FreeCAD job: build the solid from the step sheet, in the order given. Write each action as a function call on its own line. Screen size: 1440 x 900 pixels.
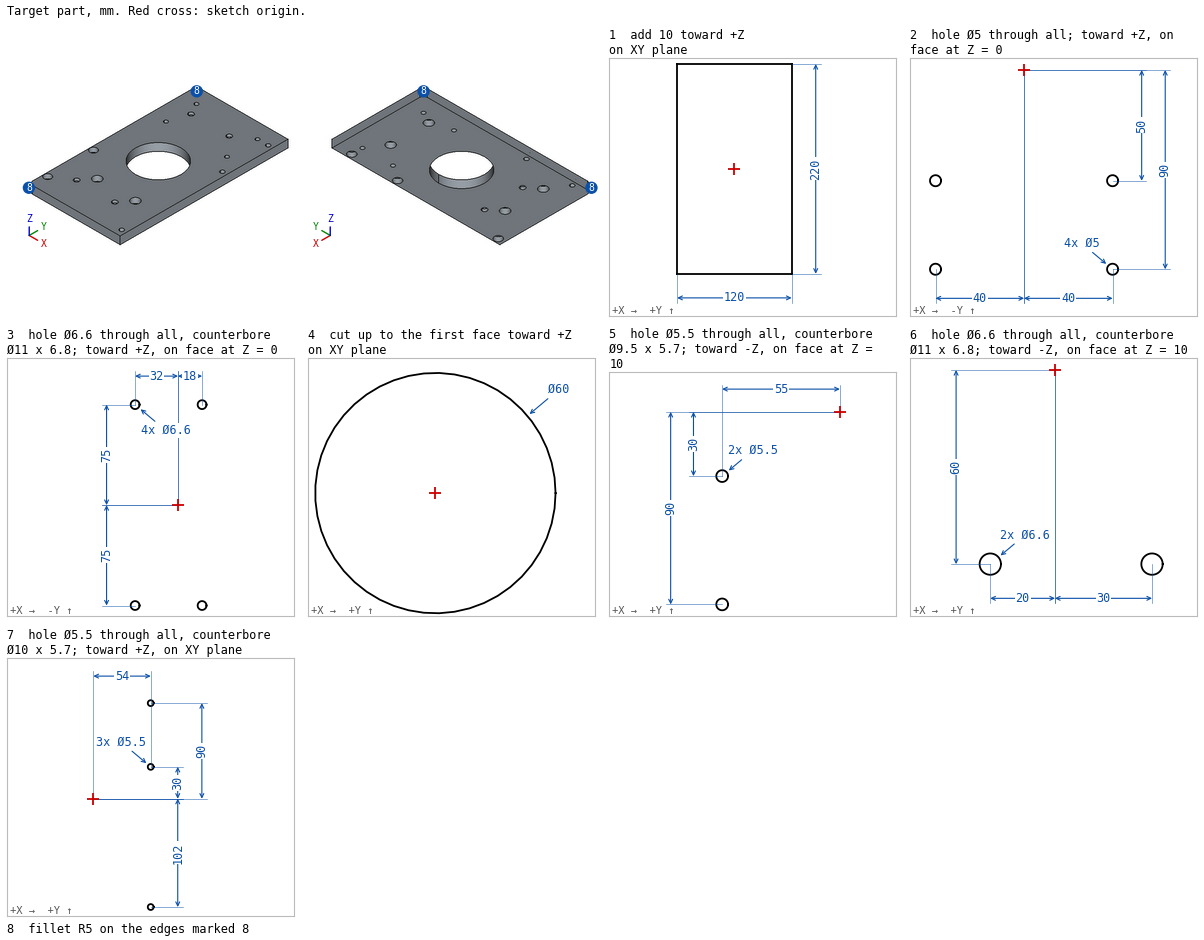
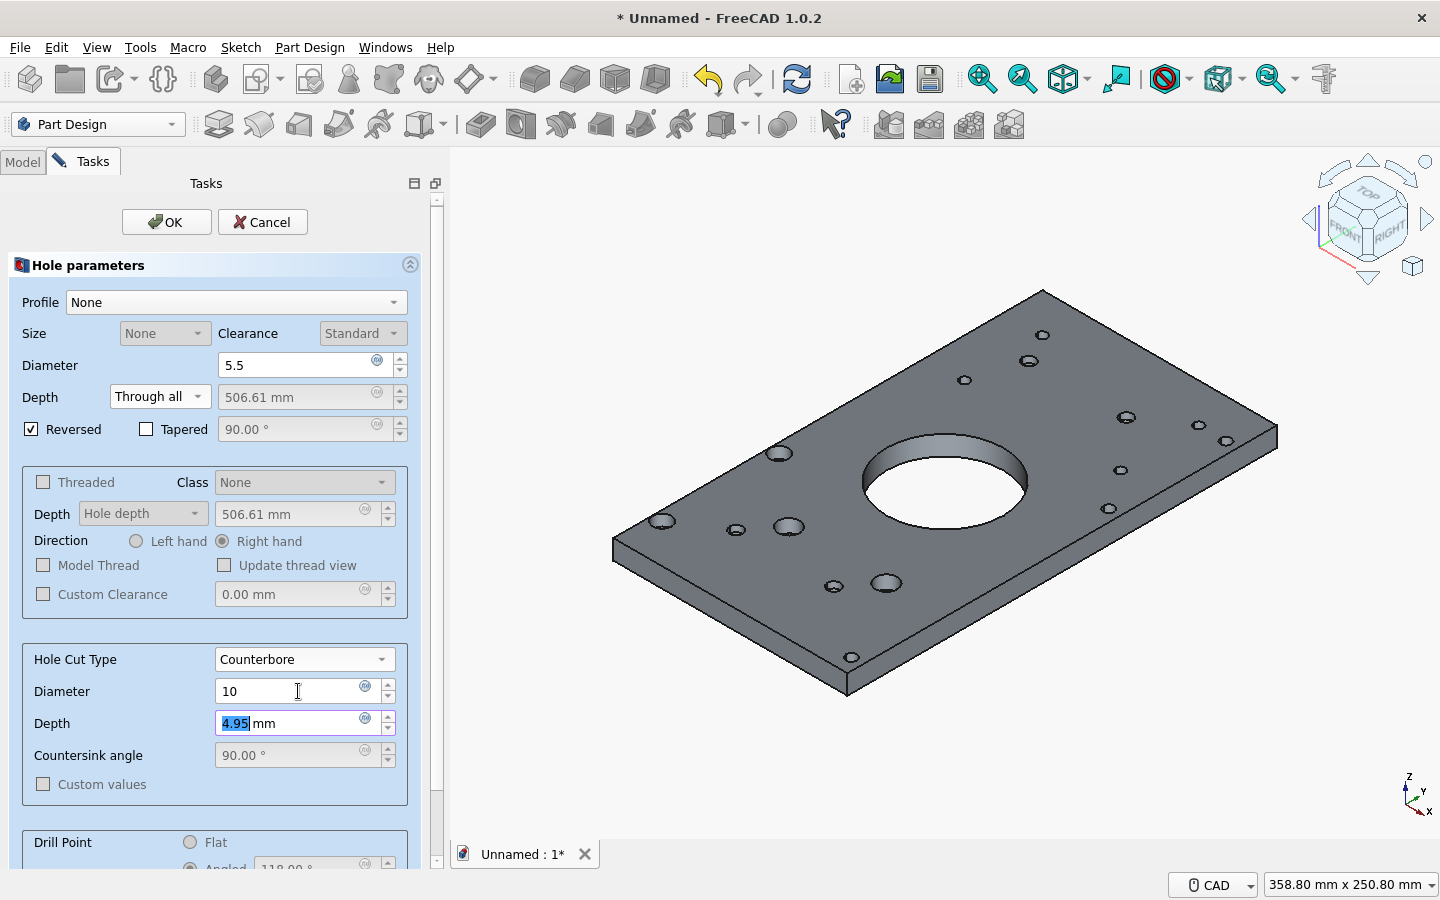
text(5.7)
key(Tab)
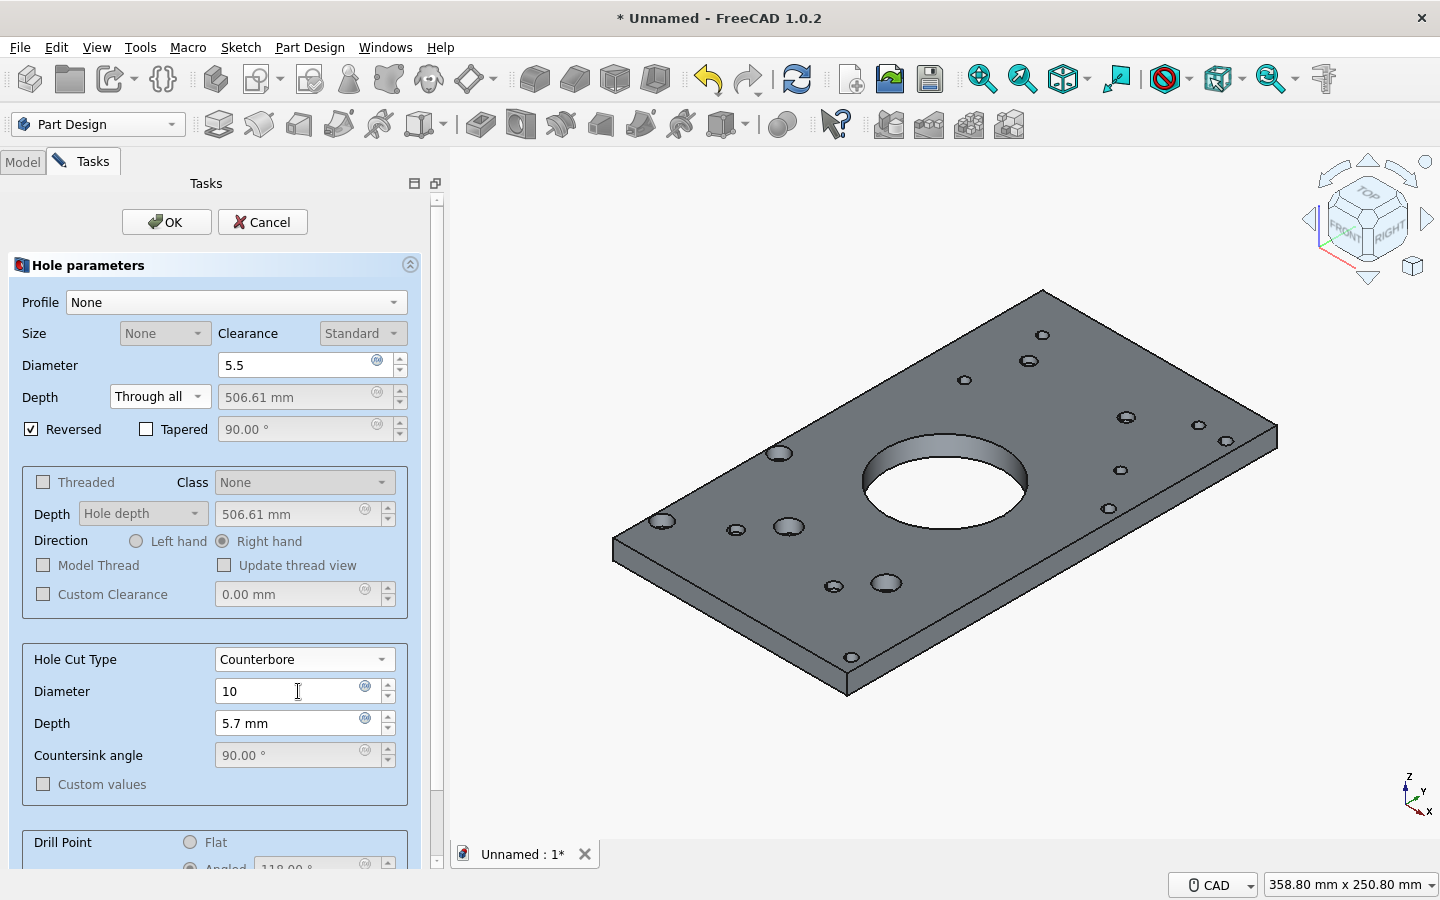
click(167, 222)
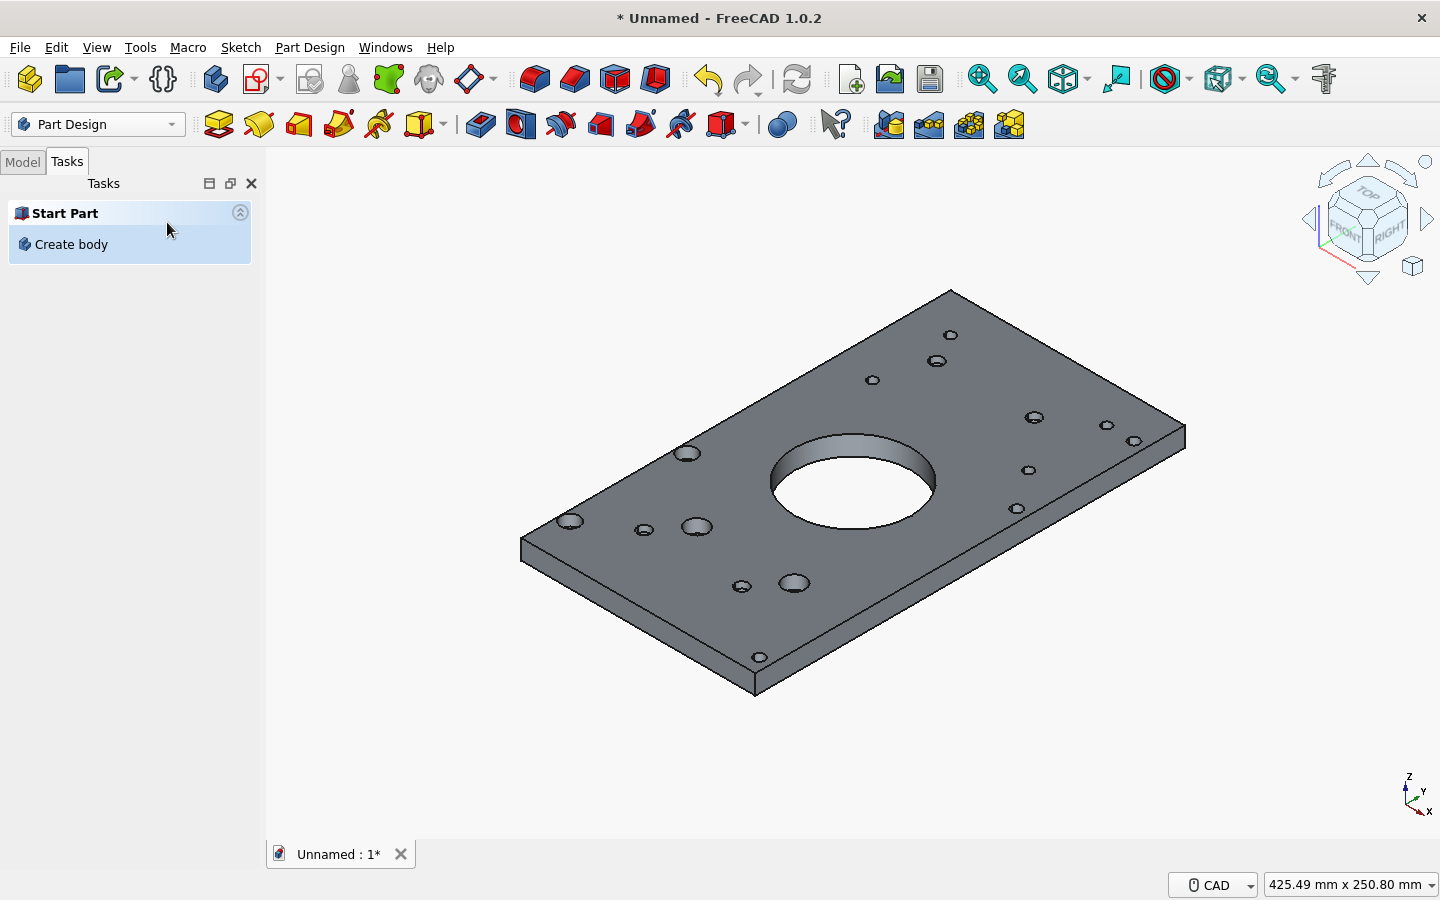
key(2)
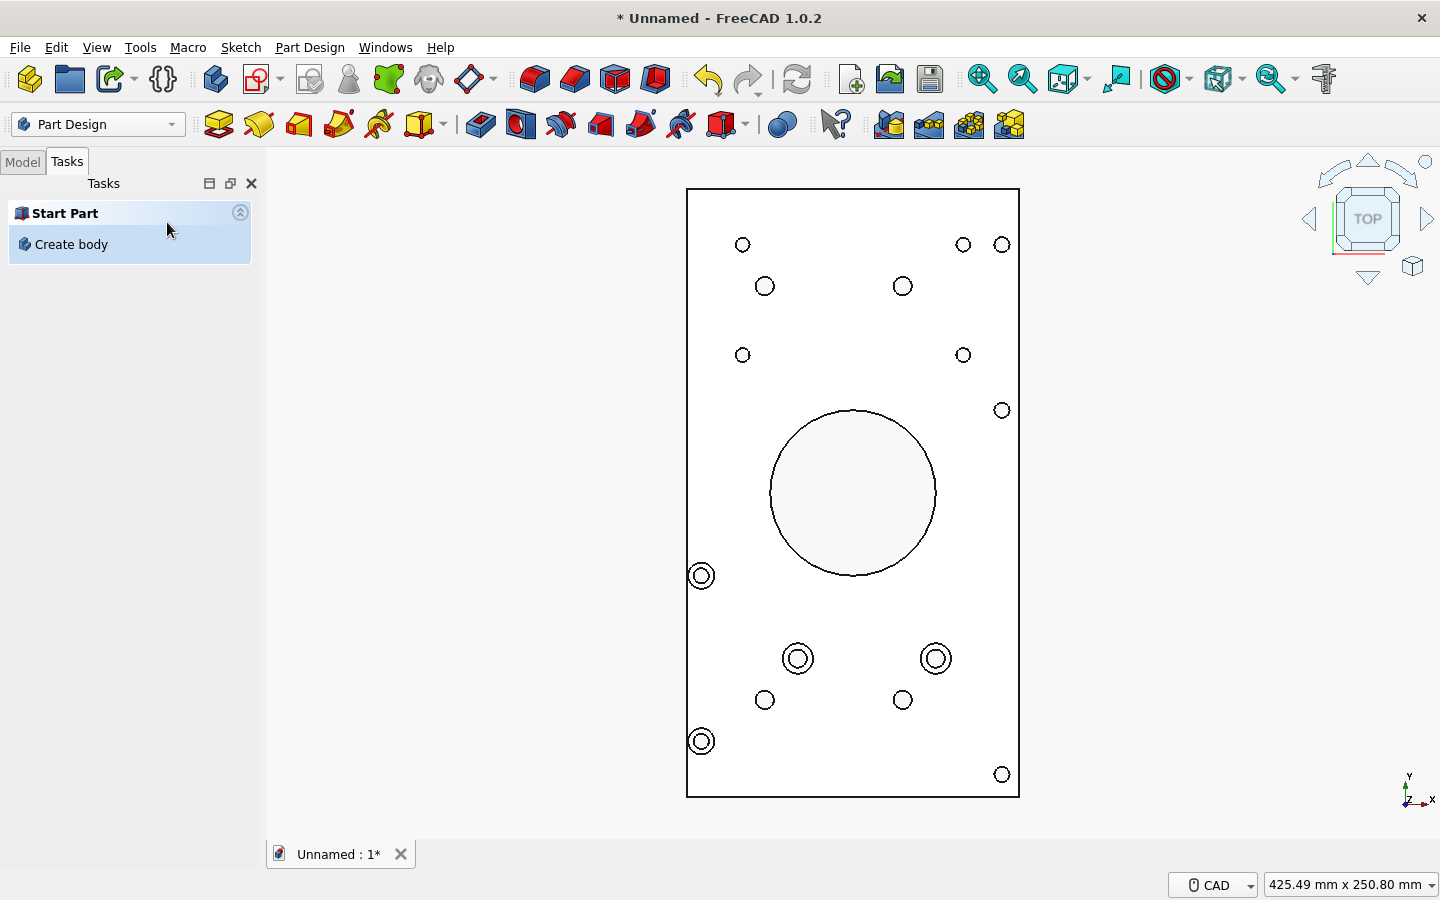
key(0)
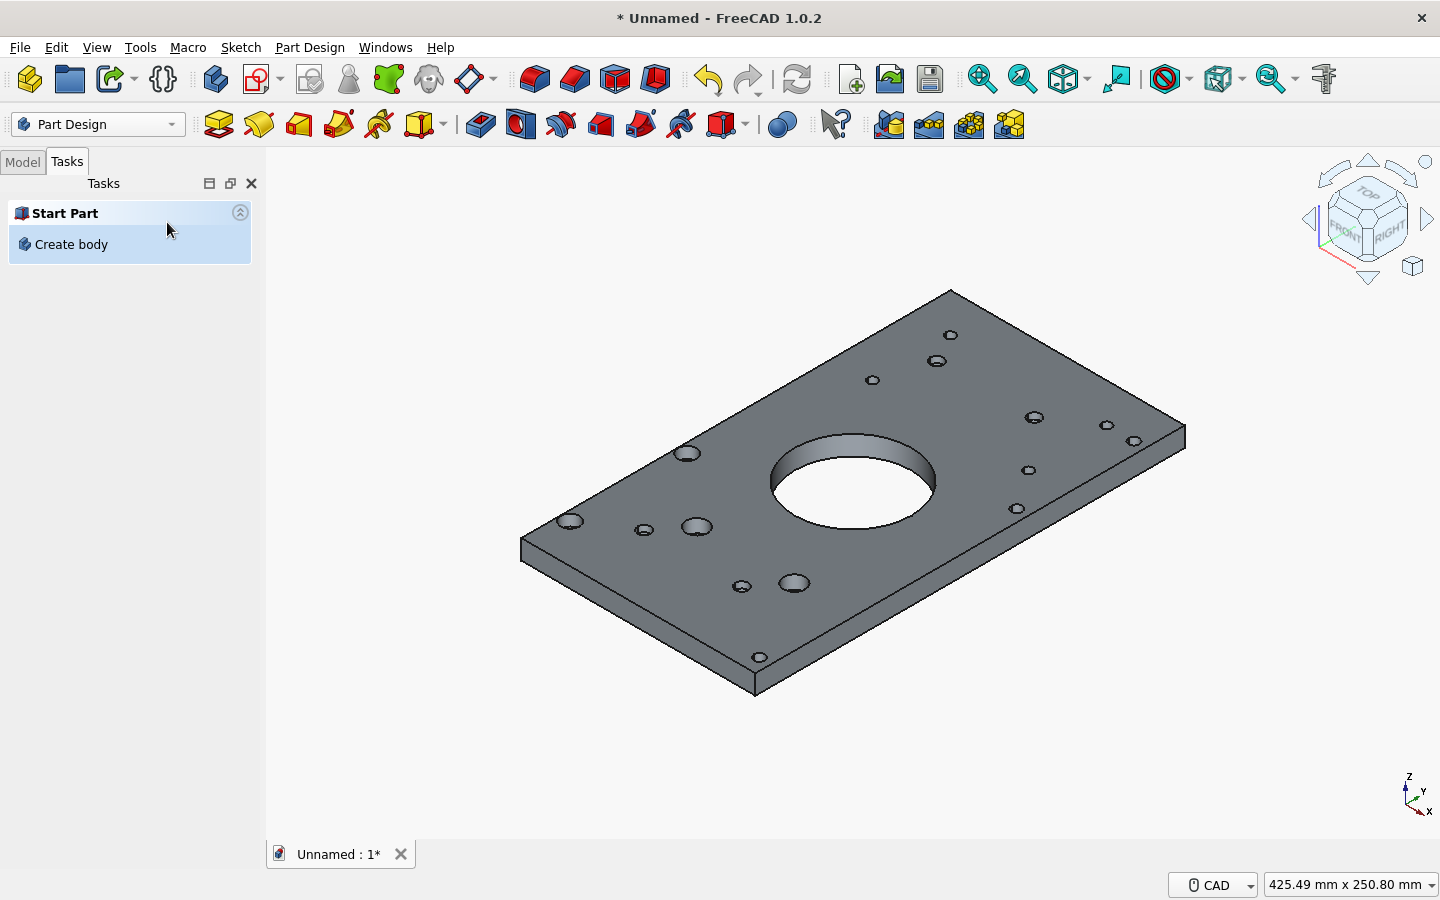
key(1)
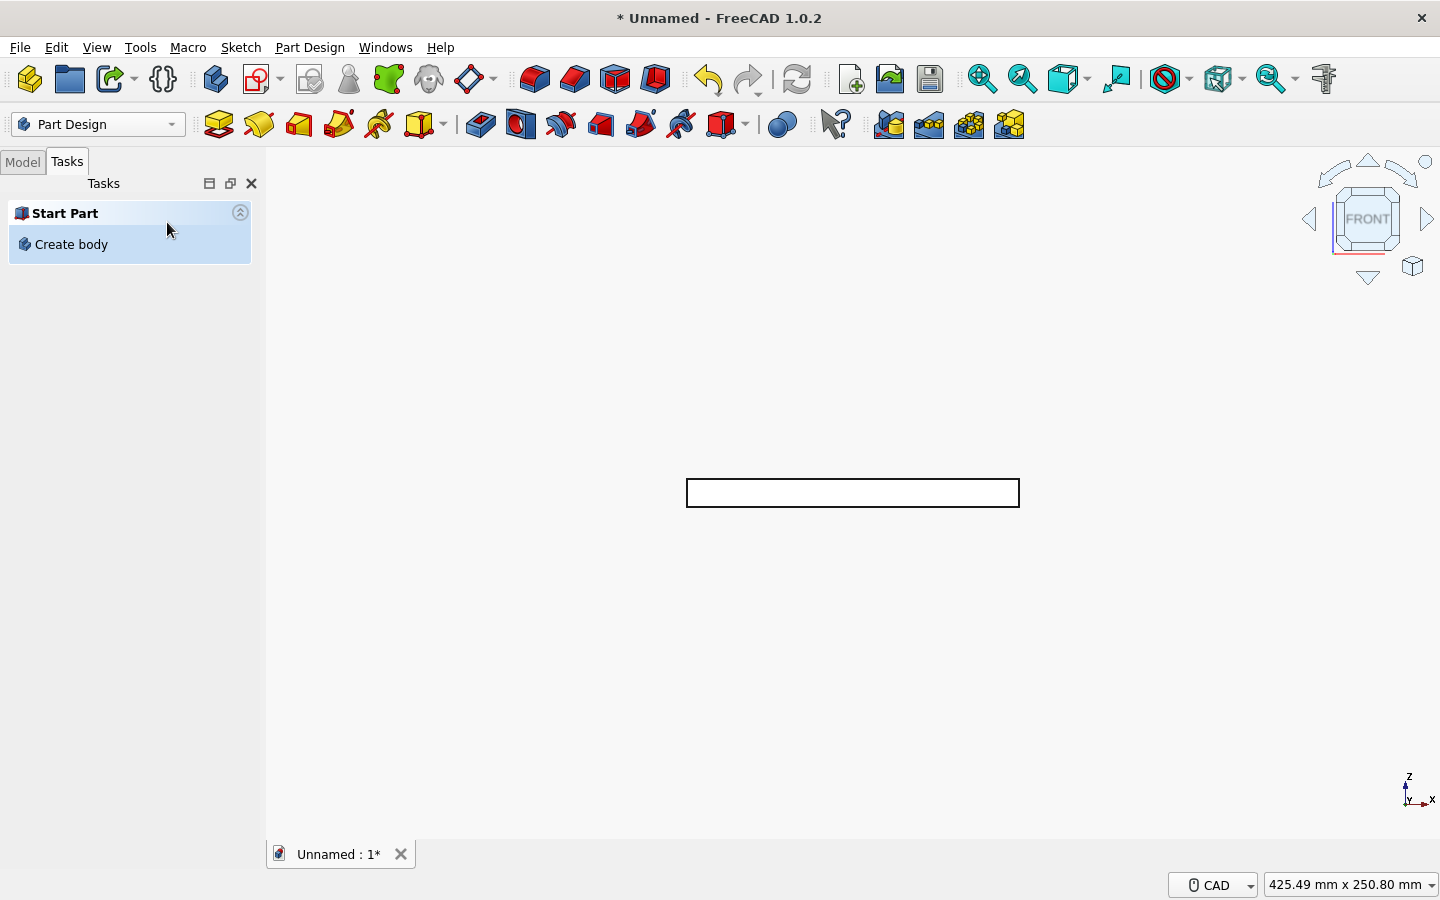
key(v)
key(f)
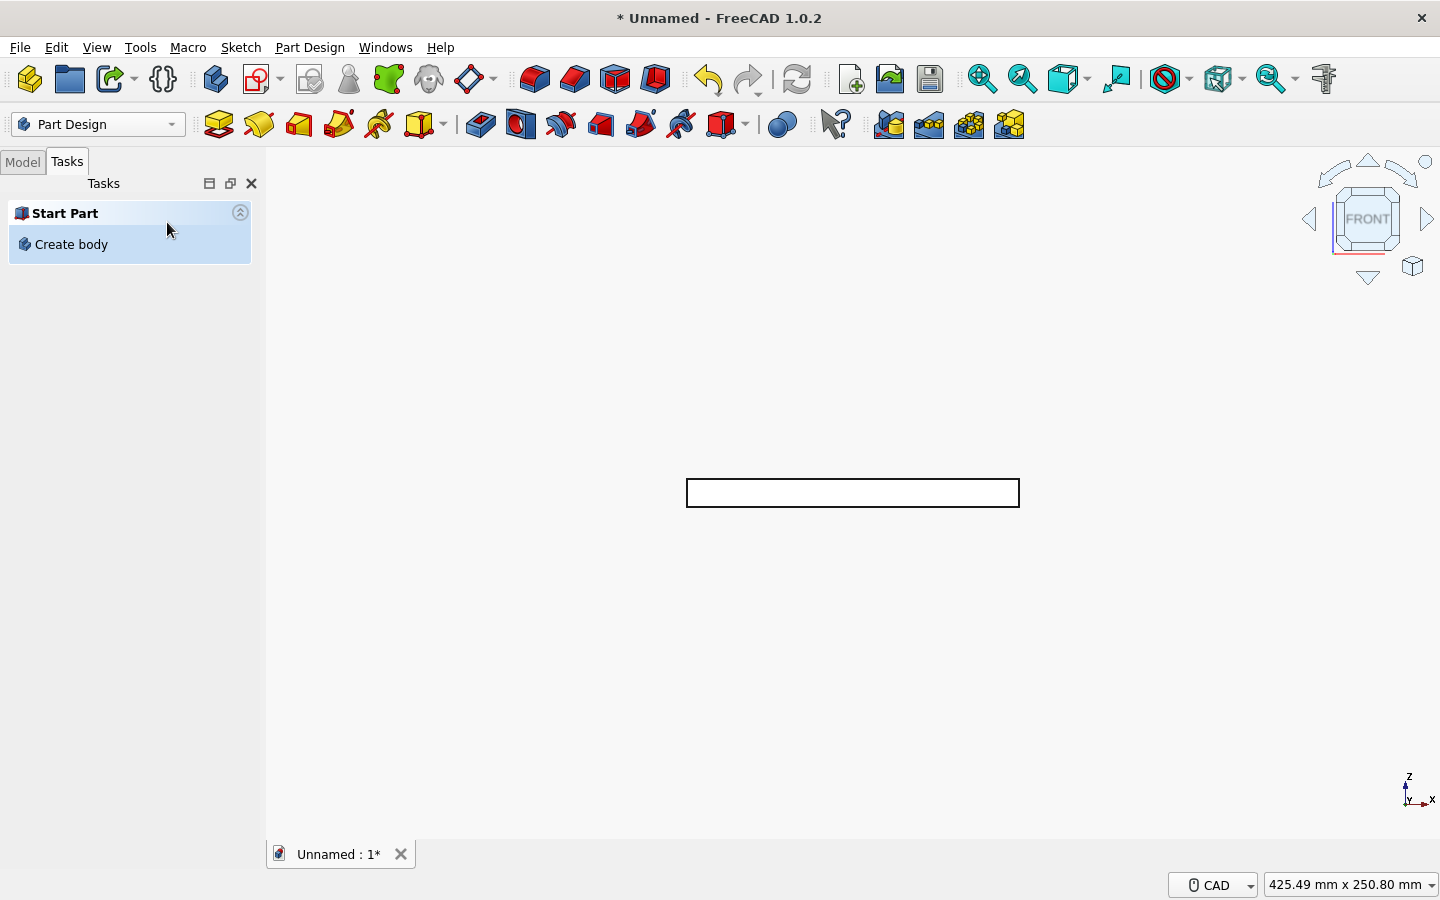
click(687, 492)